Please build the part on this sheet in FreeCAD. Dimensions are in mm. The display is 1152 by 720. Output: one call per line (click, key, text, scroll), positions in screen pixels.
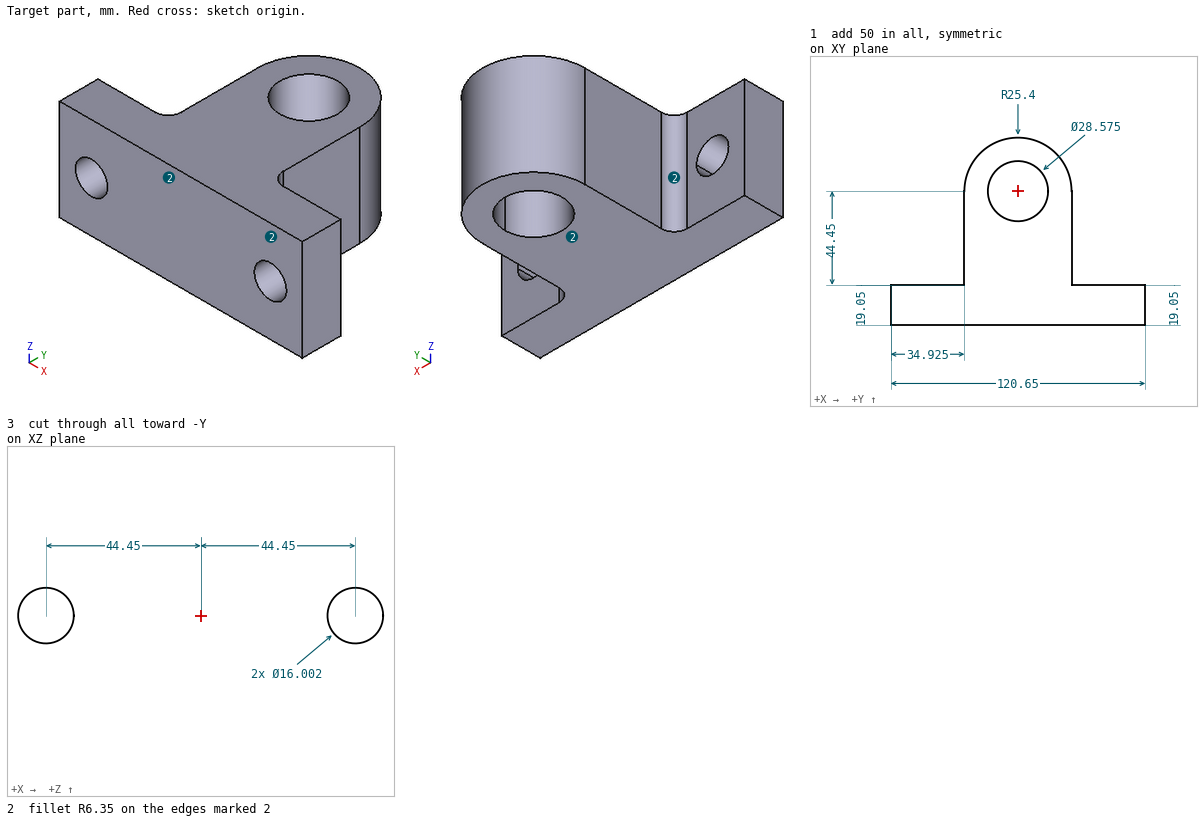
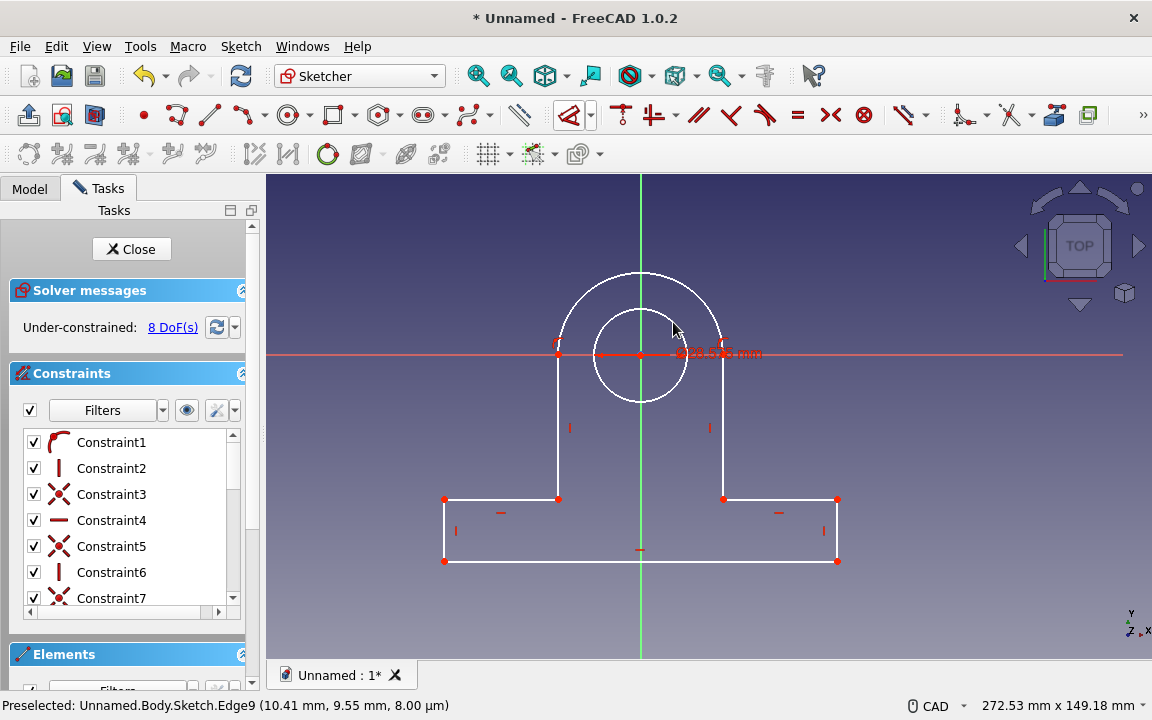
drag(630, 345, 651, 365)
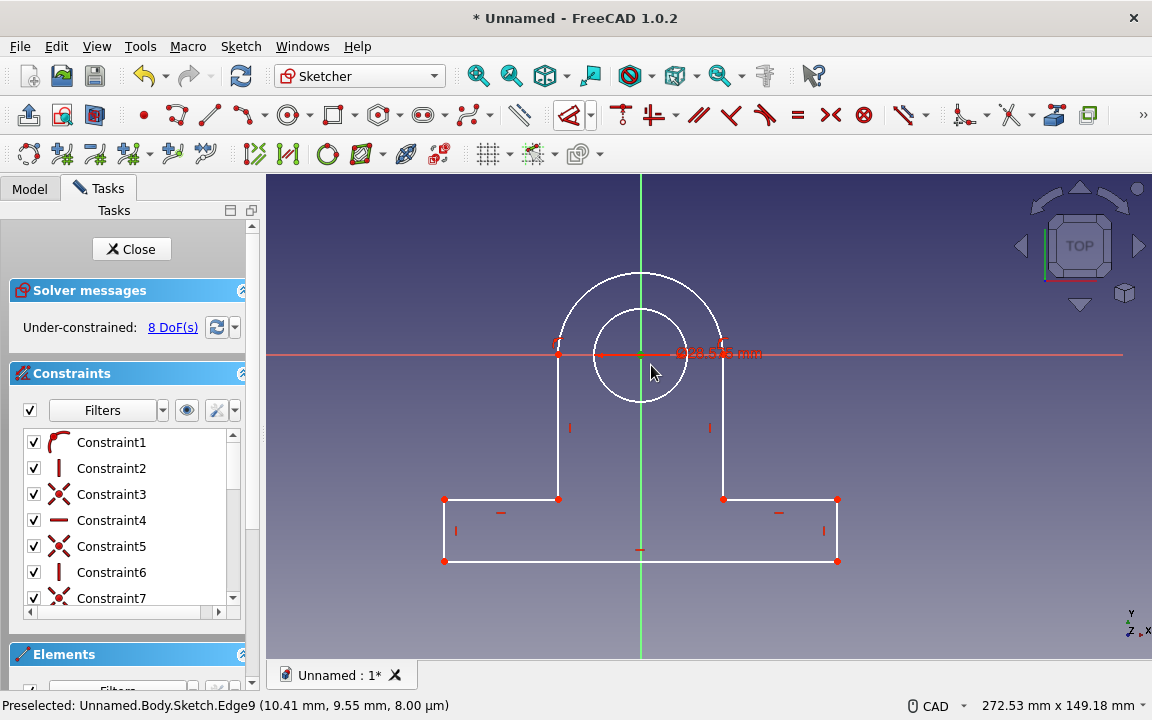
click(621, 116)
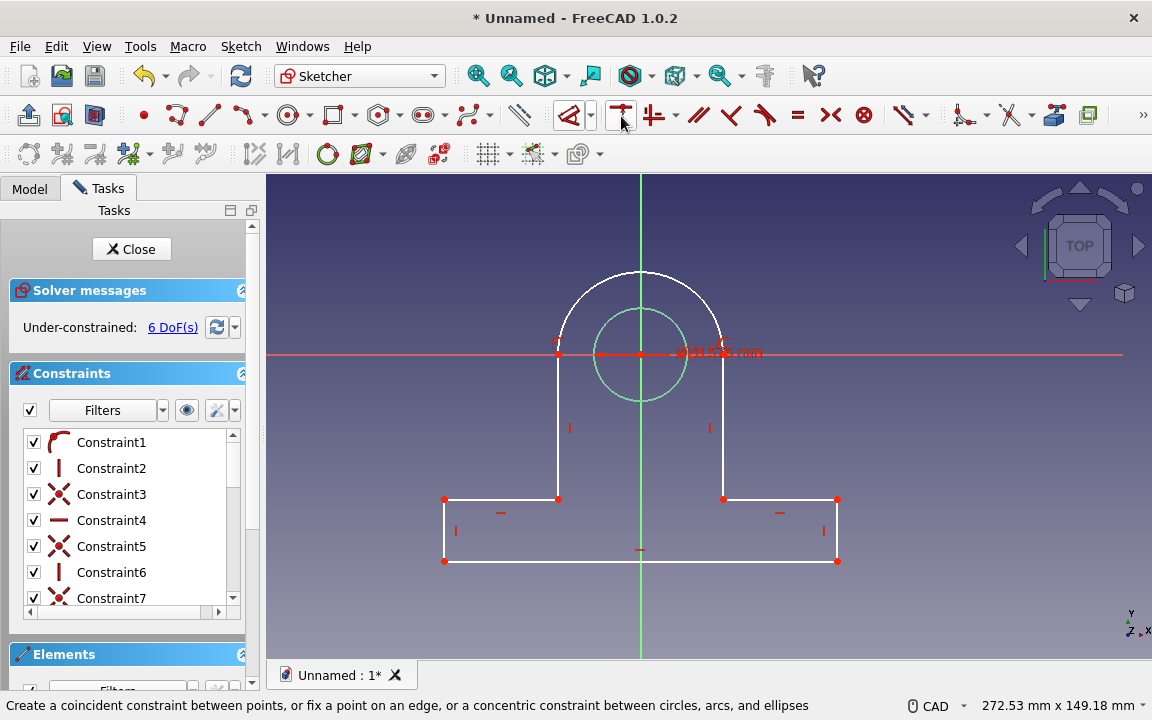
click(568, 116)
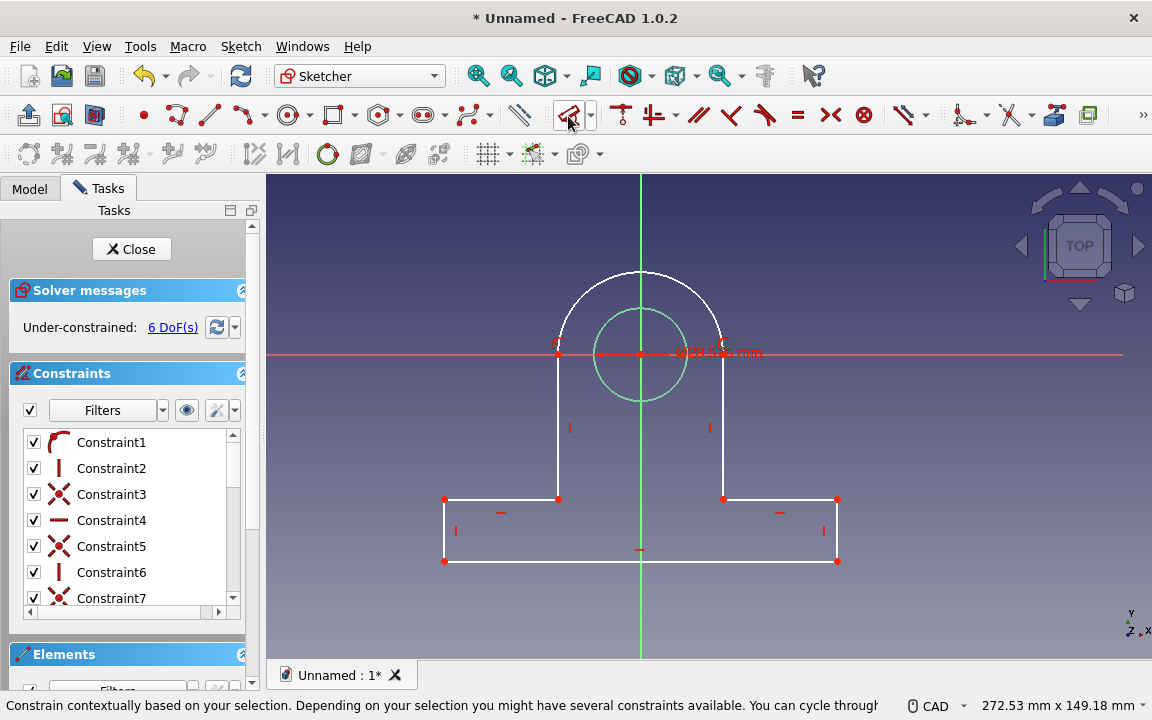
click(689, 288)
click(708, 262)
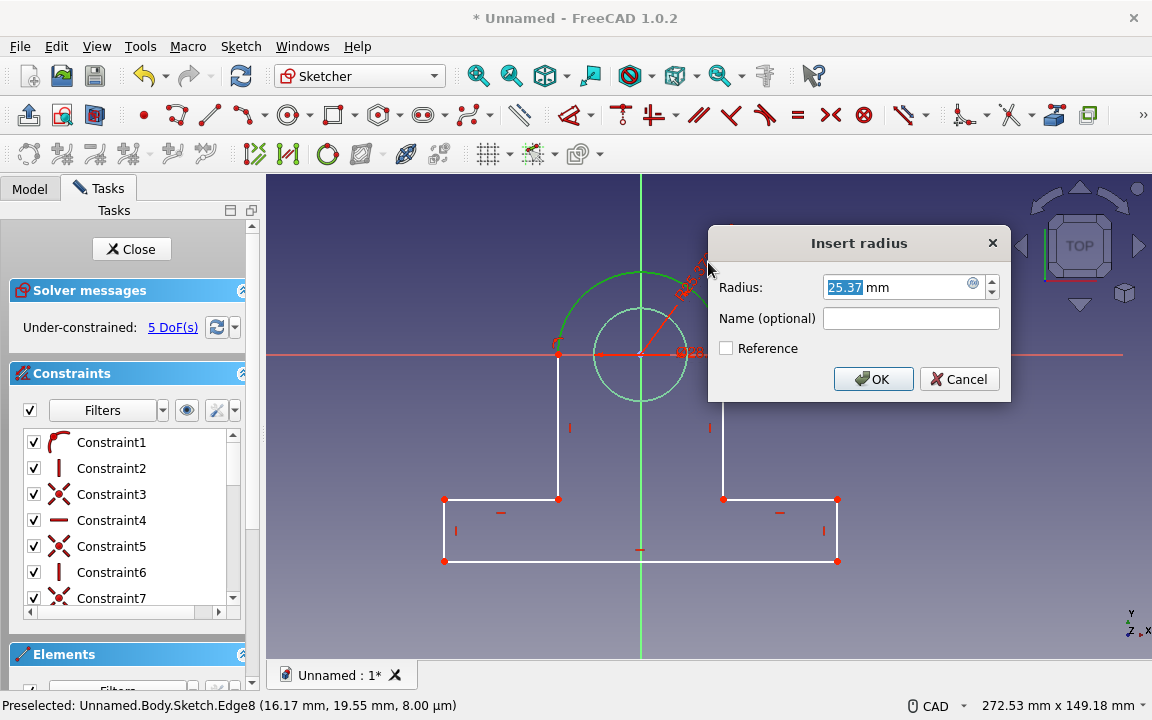
text(25.4)
key(Return)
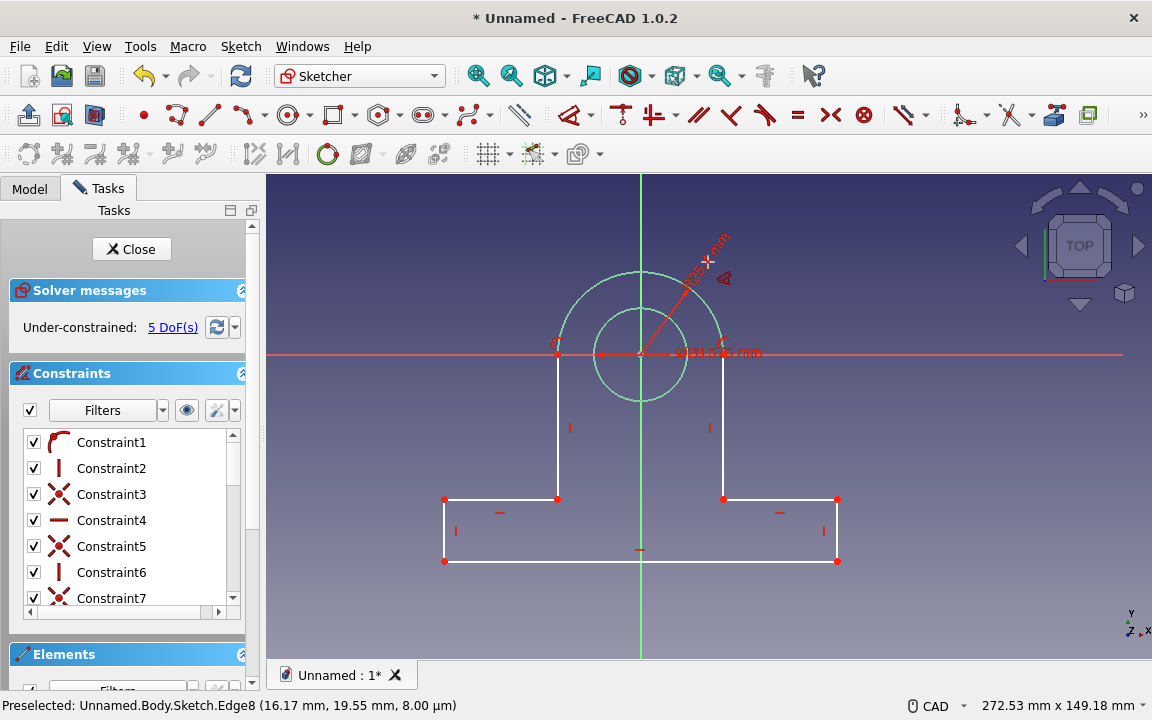
click(558, 398)
click(524, 427)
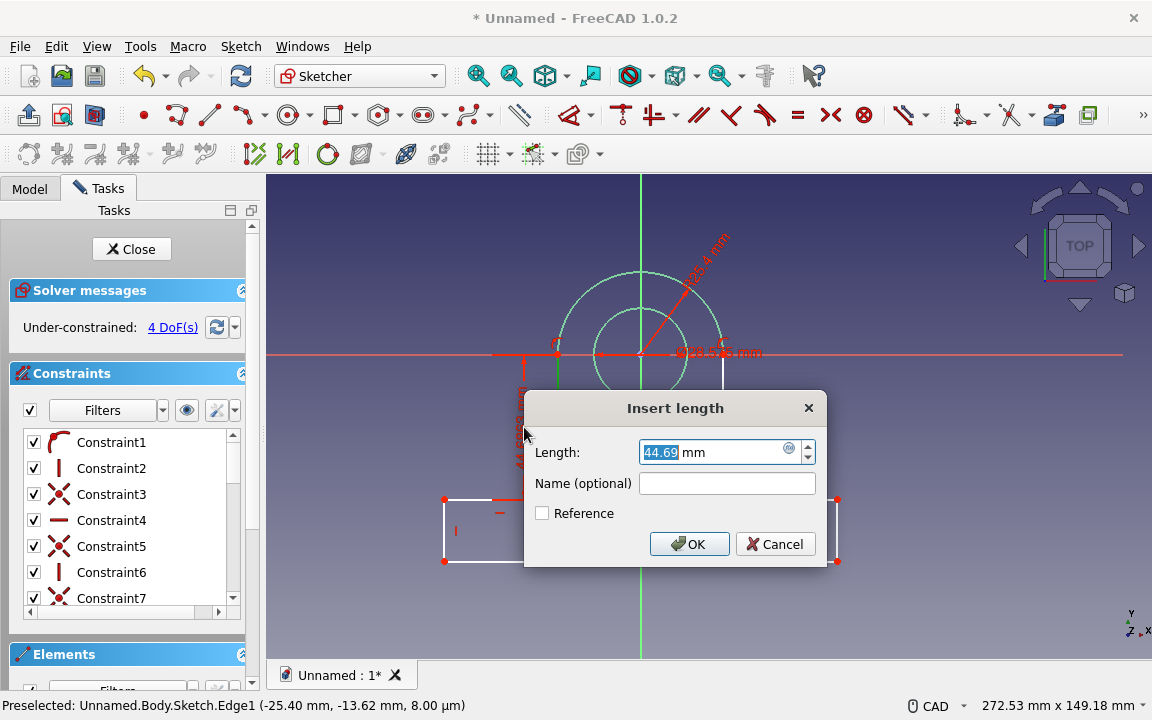
text(44.45)
key(Return)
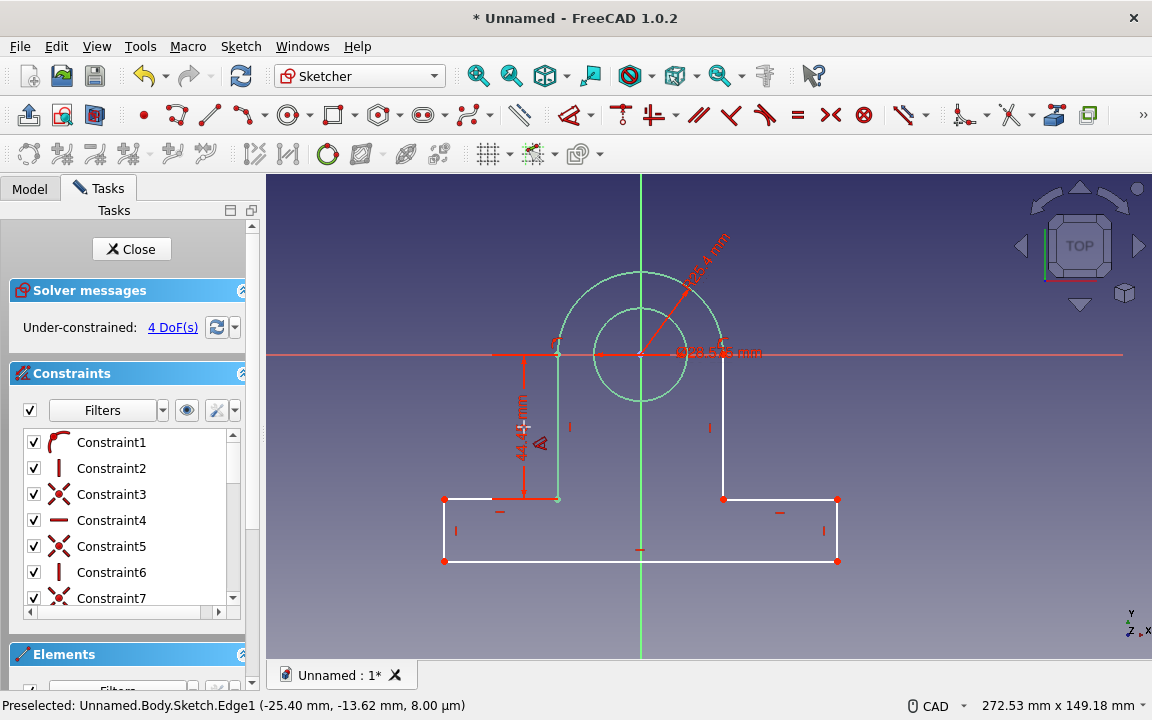
click(444, 518)
click(410, 531)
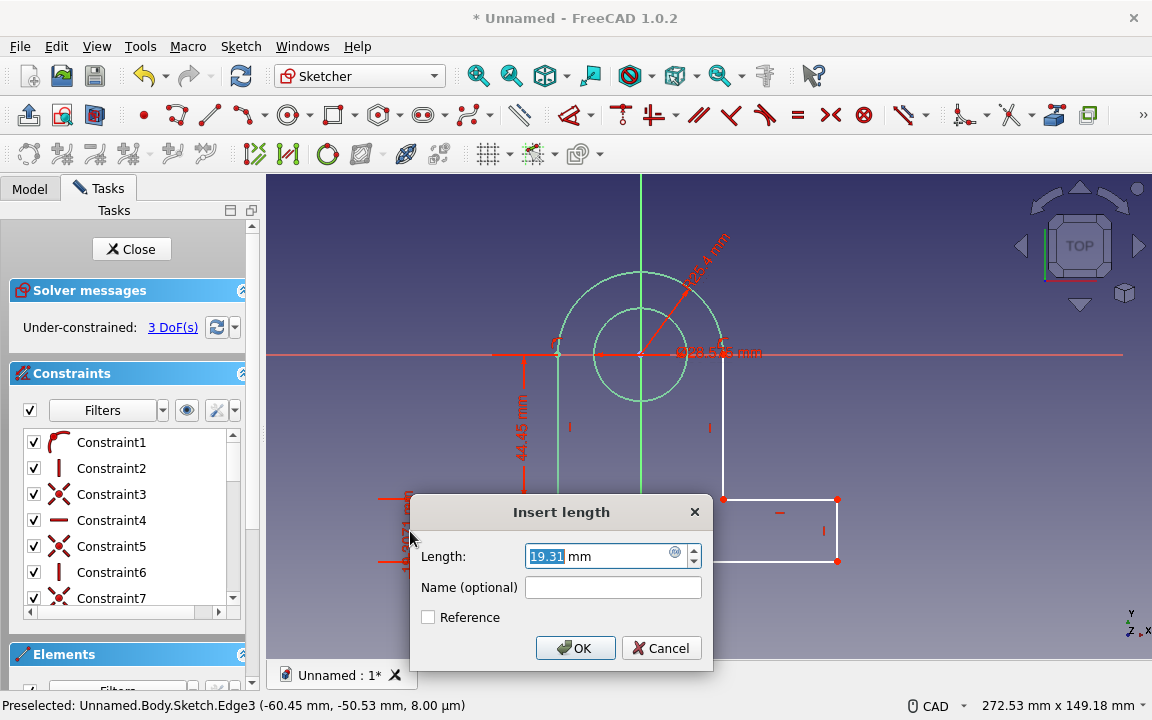
text(19.05)
key(Return)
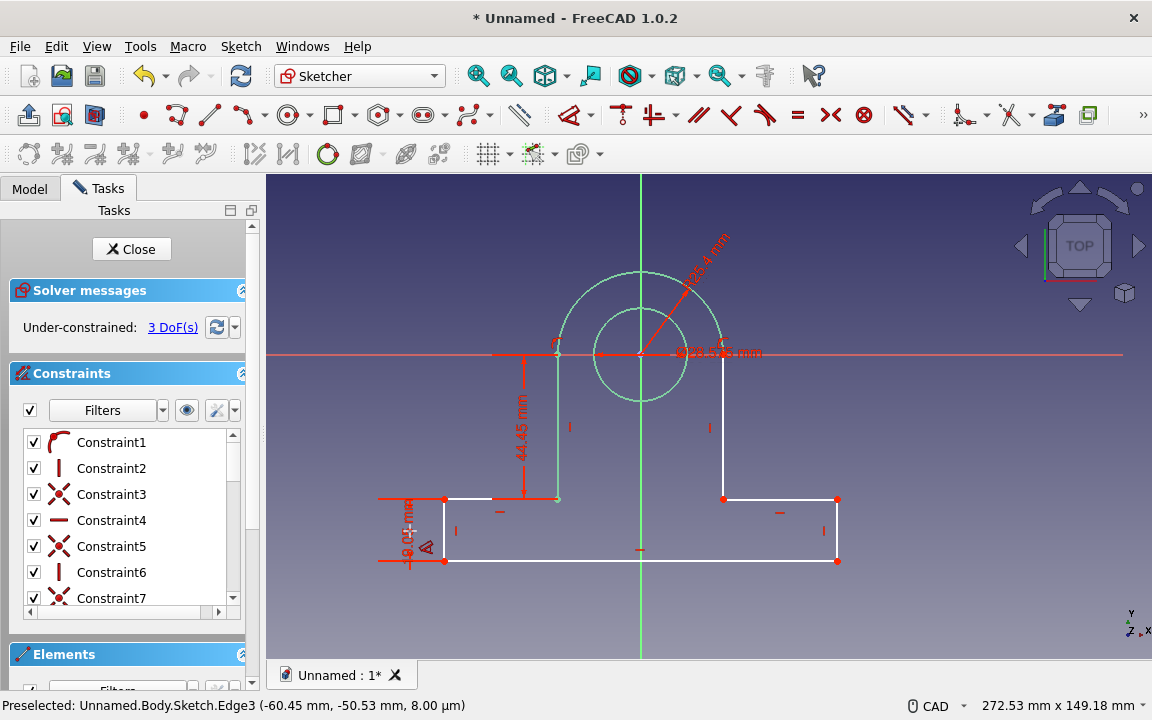
click(837, 543)
click(871, 531)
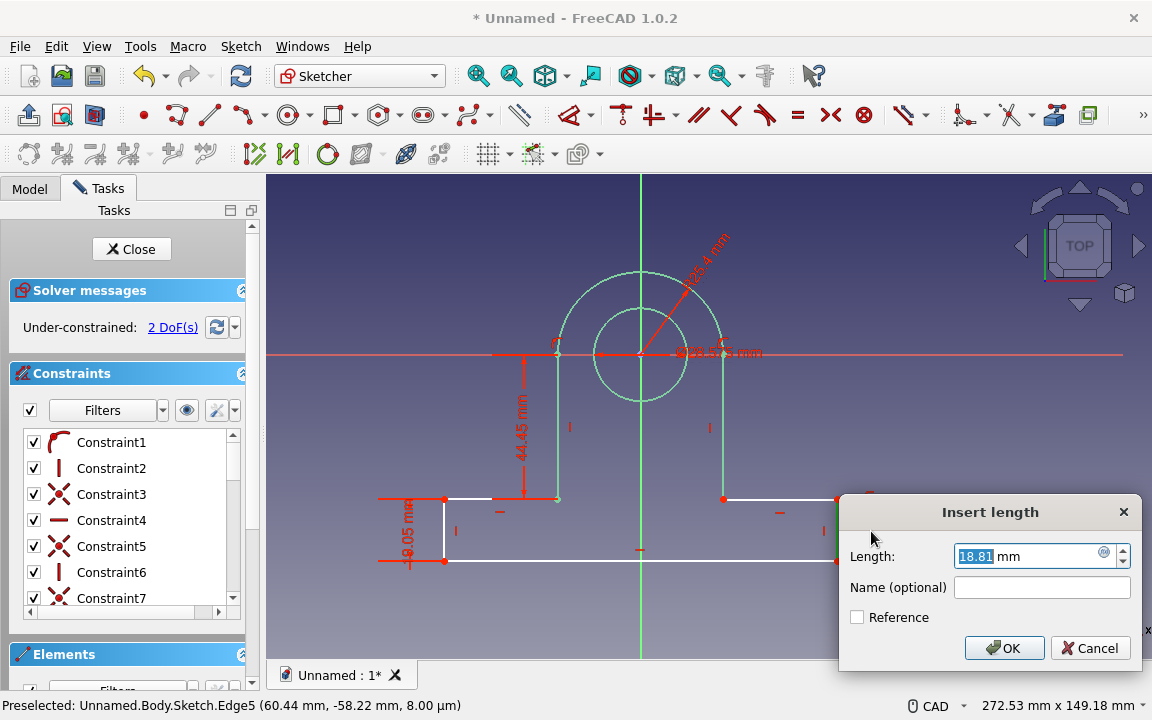
text(19.05)
key(Return)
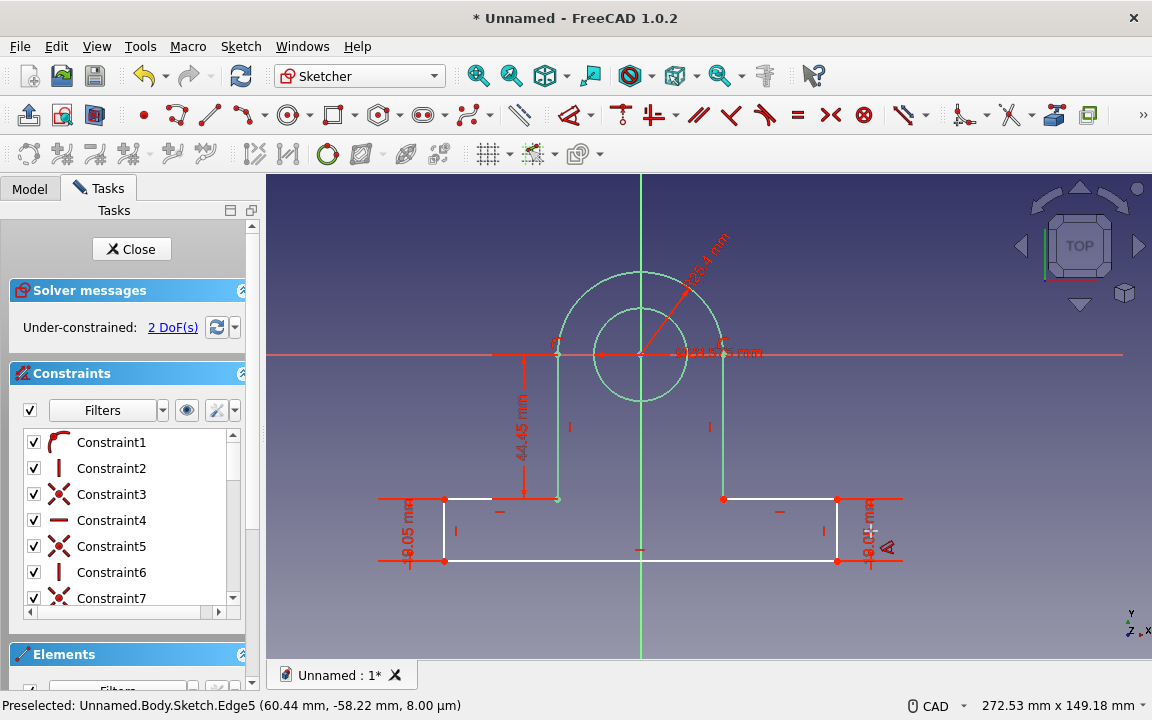
click(524, 499)
click(501, 533)